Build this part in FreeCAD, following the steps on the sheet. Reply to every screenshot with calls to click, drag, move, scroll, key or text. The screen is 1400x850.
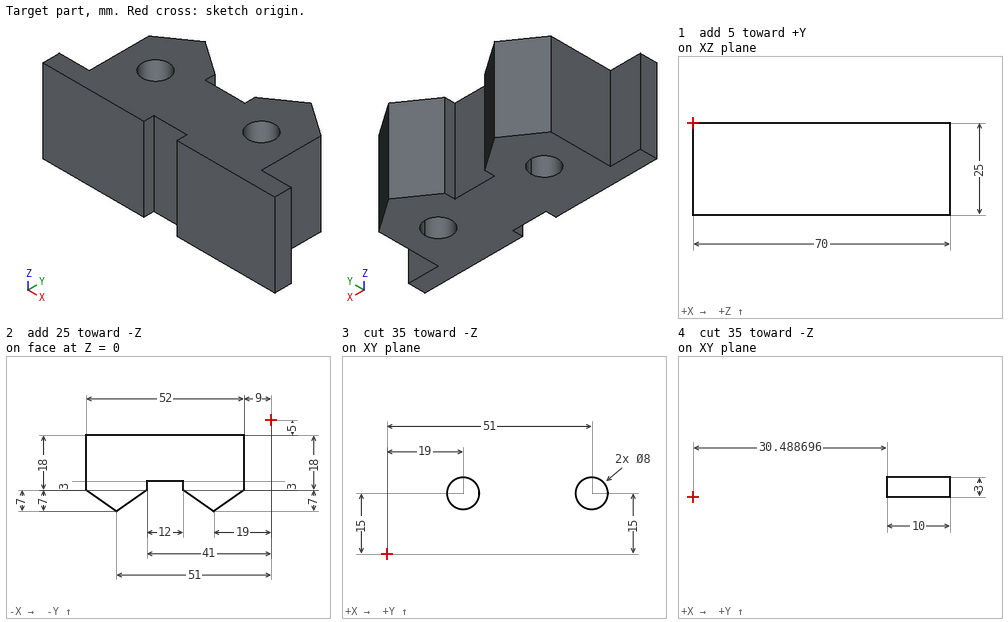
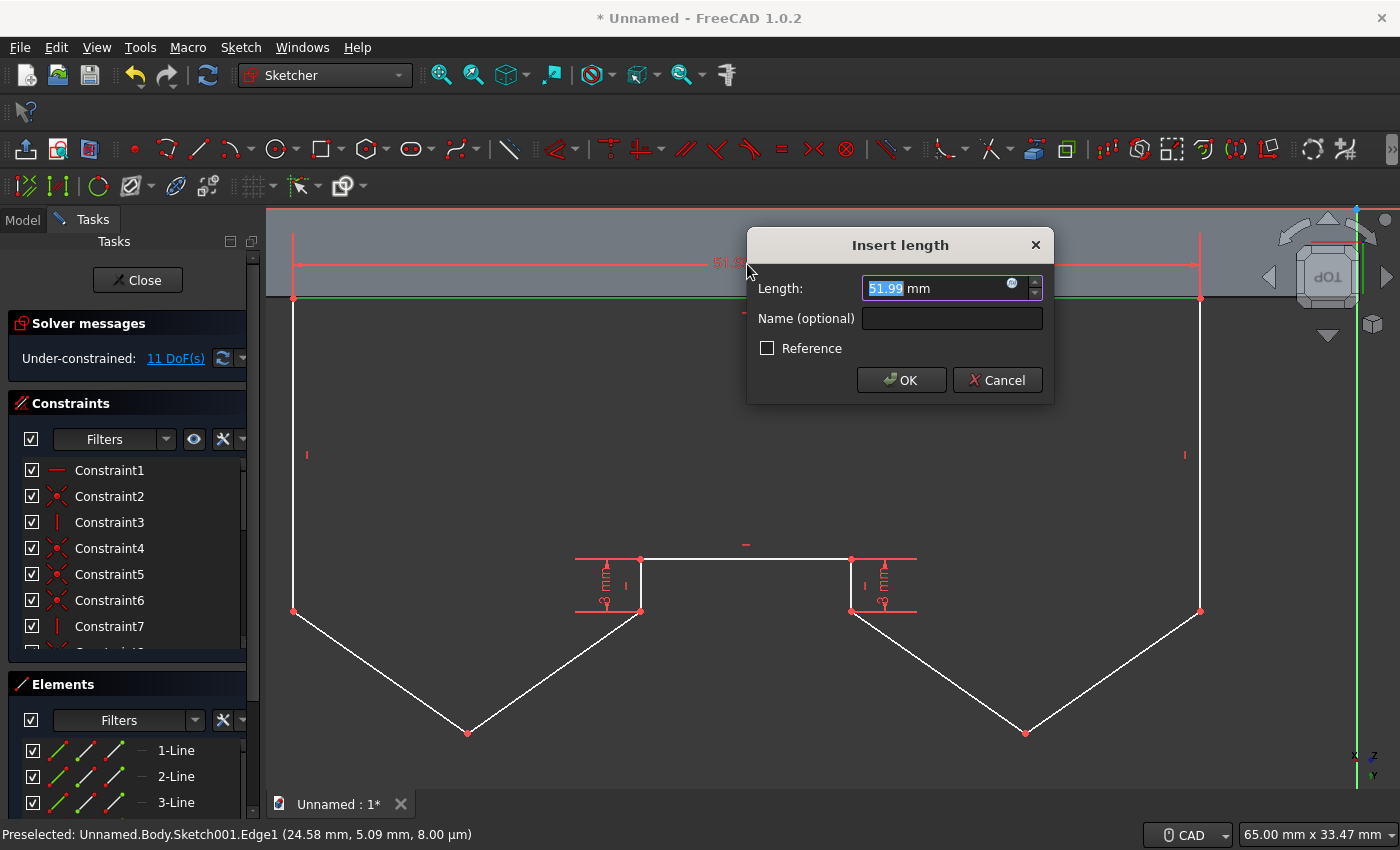
text(52)
key(Return)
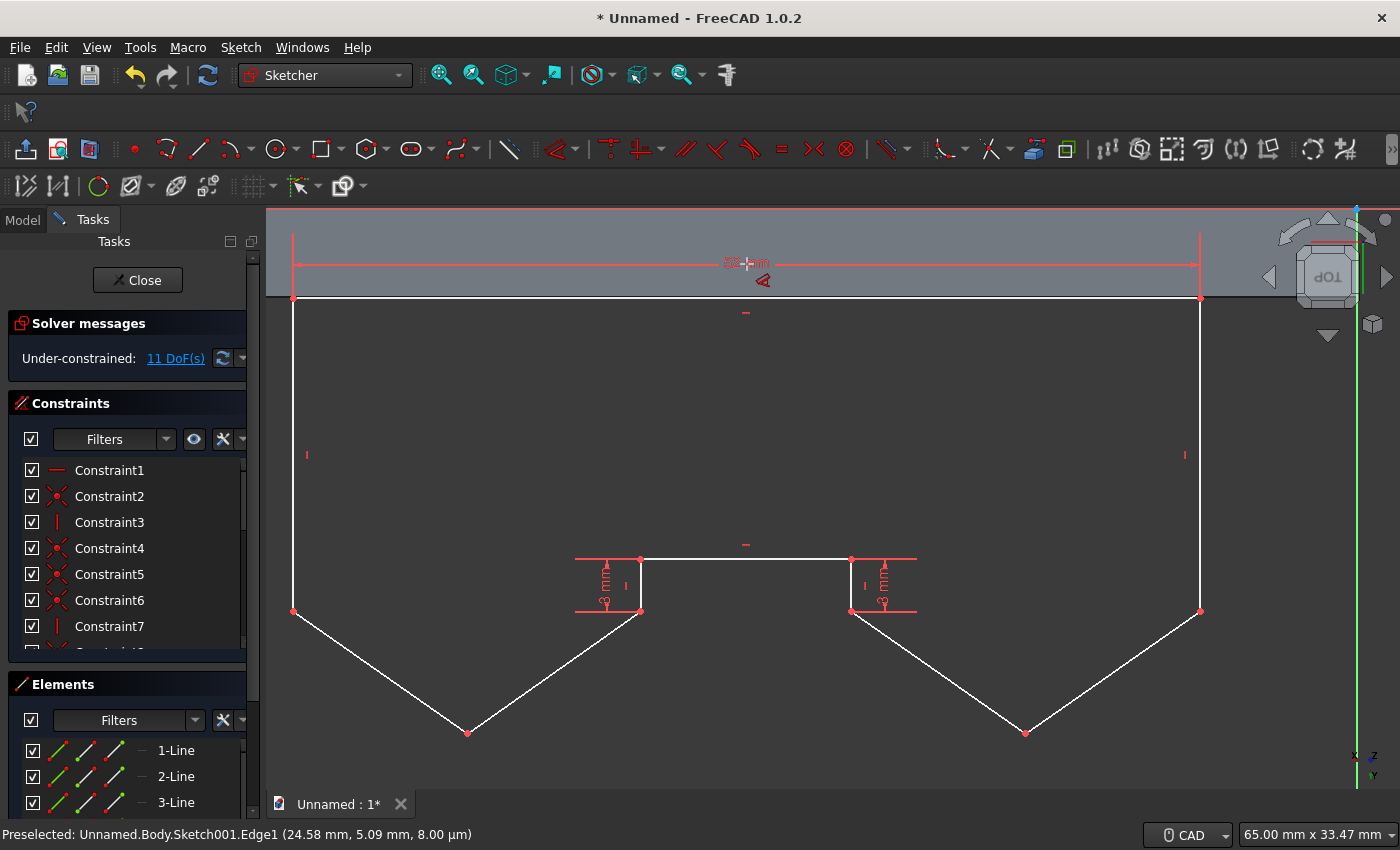
scroll(642, 550, down, 2)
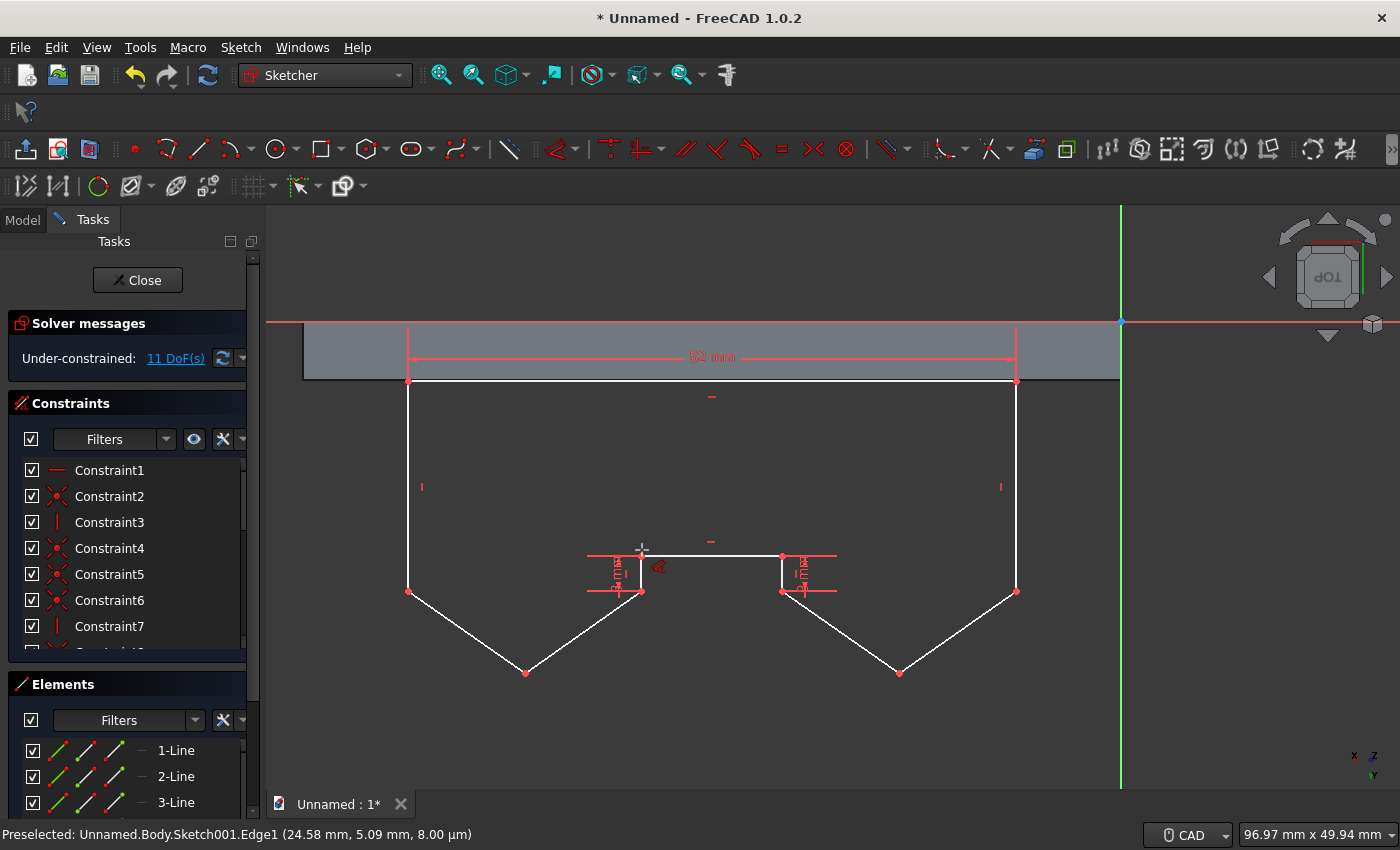
click(408, 444)
click(374, 486)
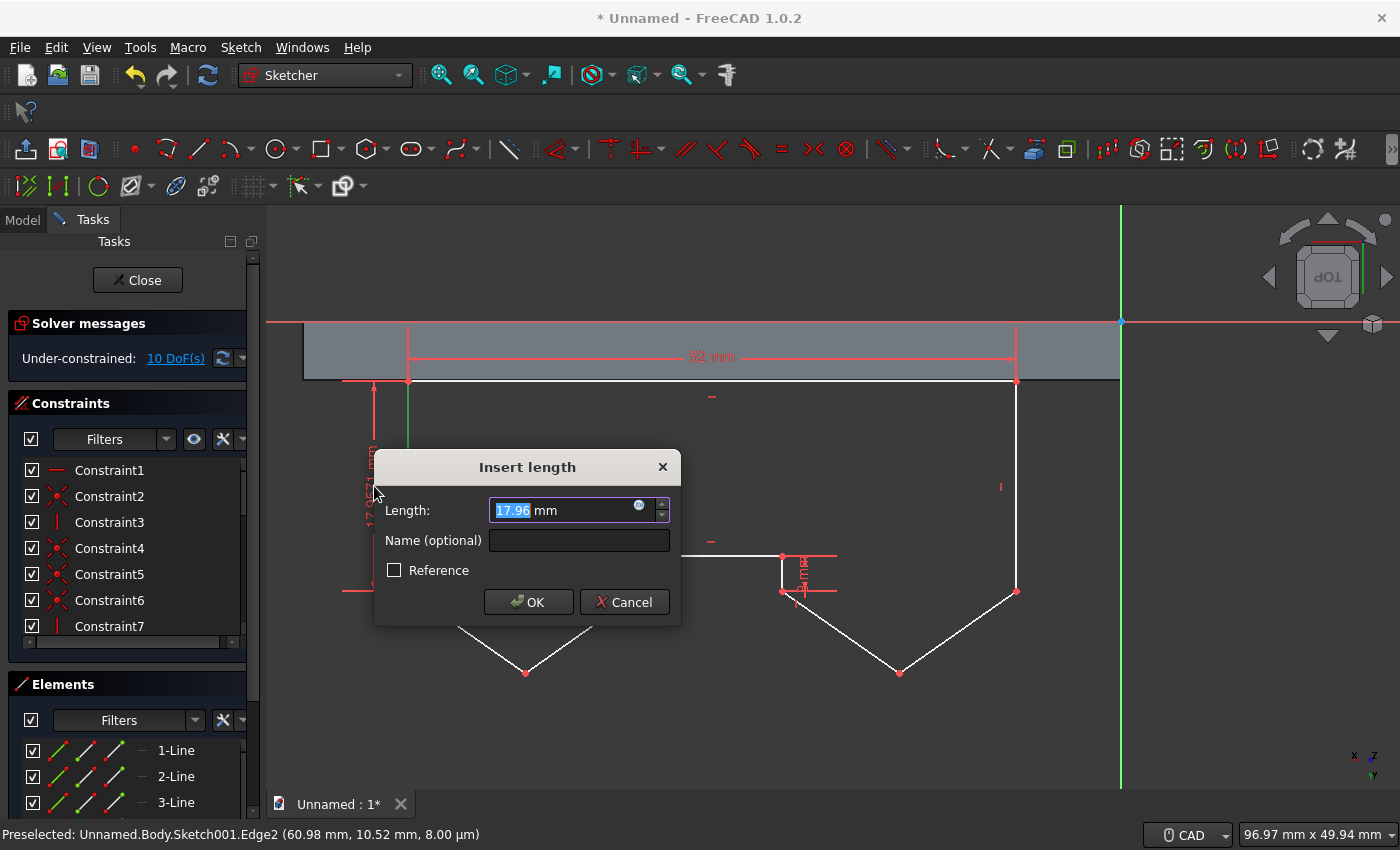
text(18)
key(Return)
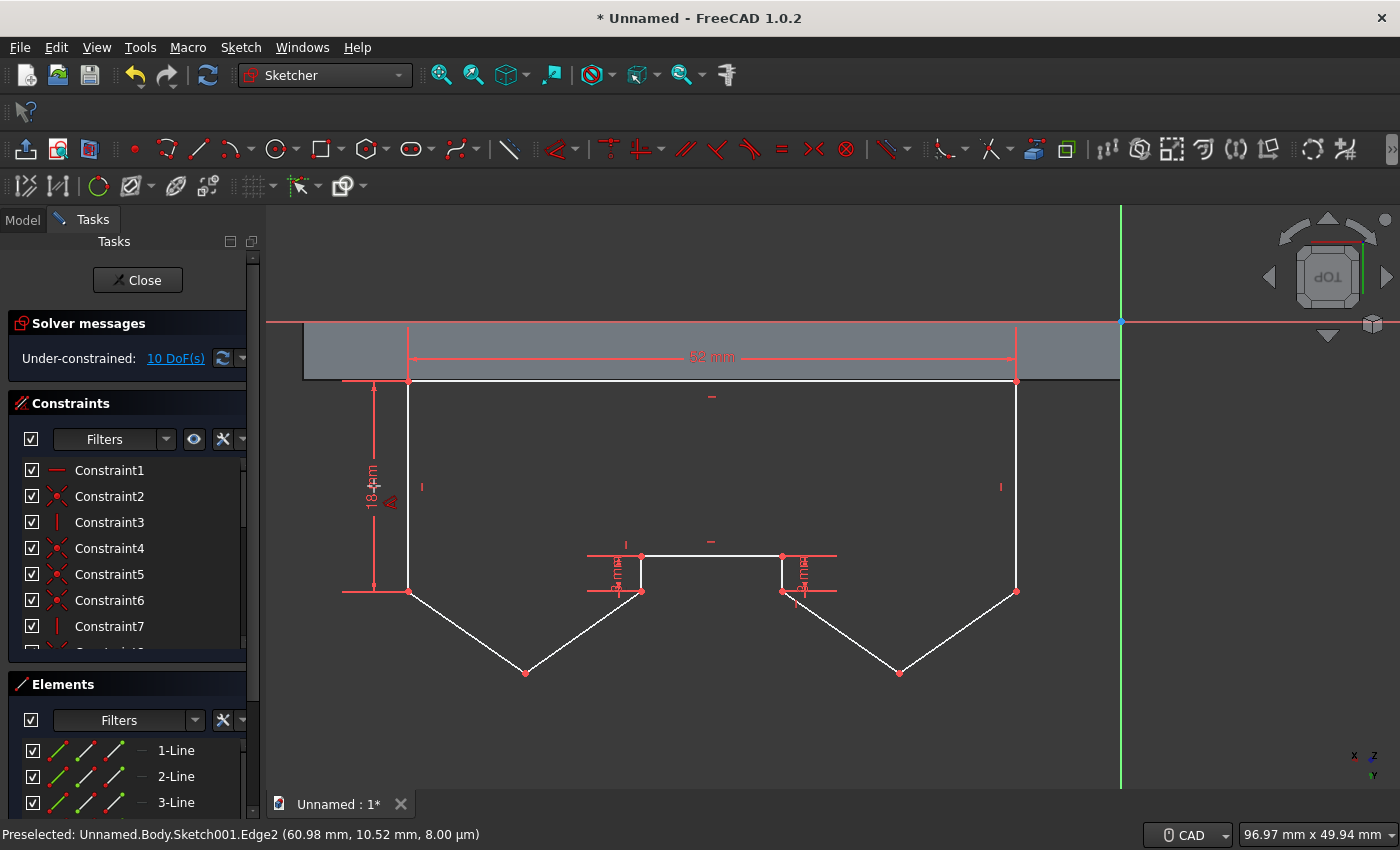
click(684, 556)
click(712, 590)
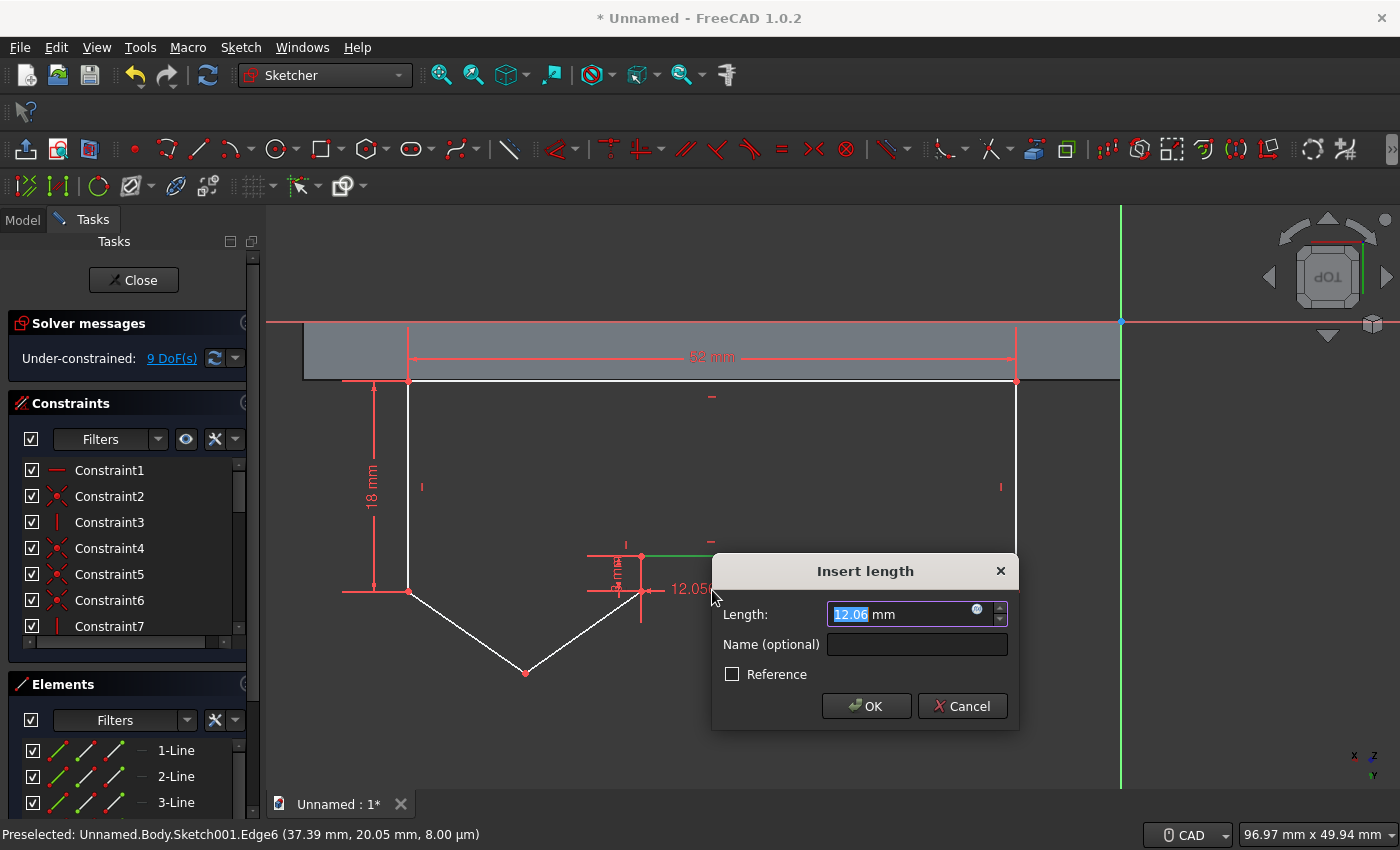
text(12)
key(Return)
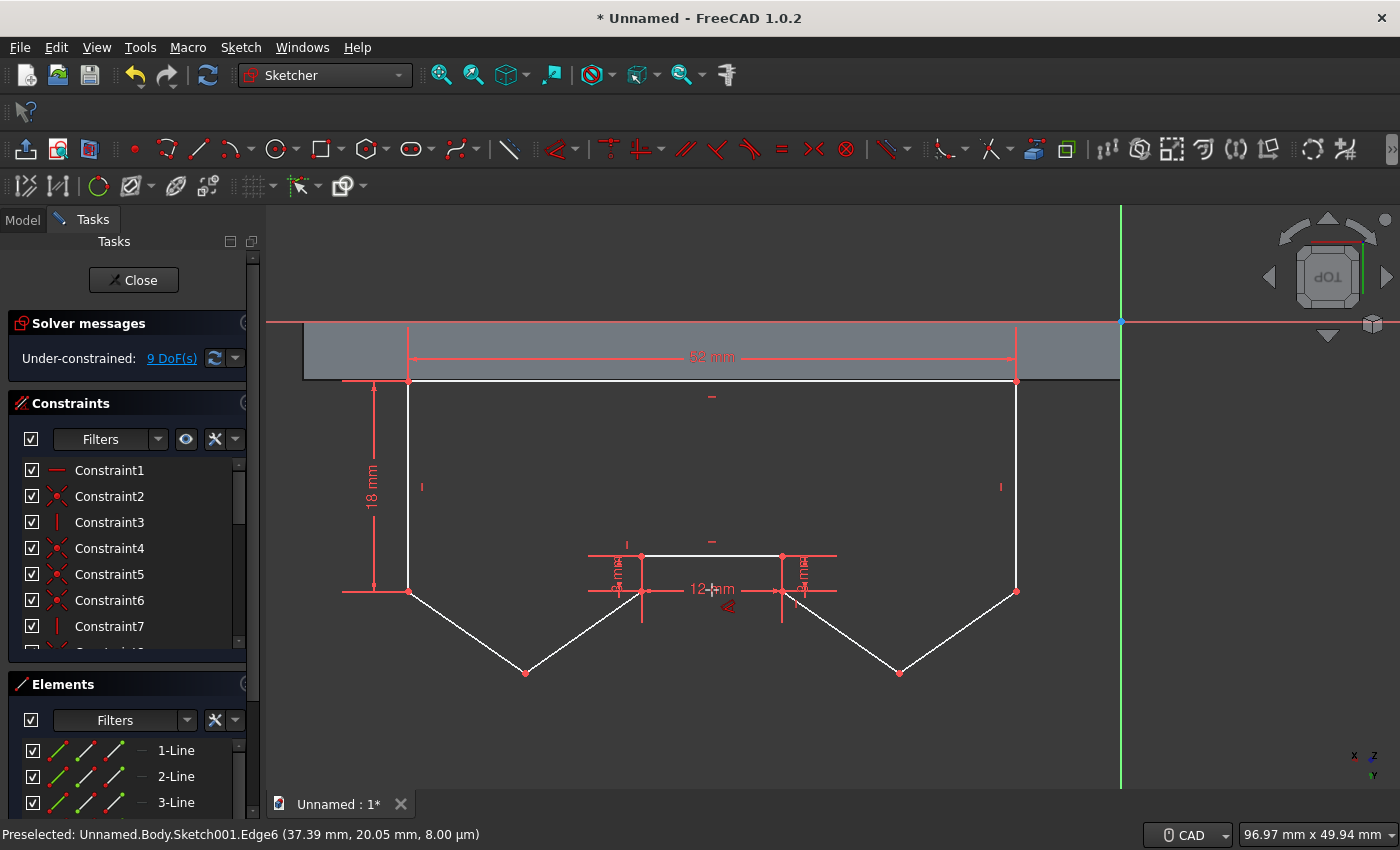
click(1016, 528)
click(1050, 486)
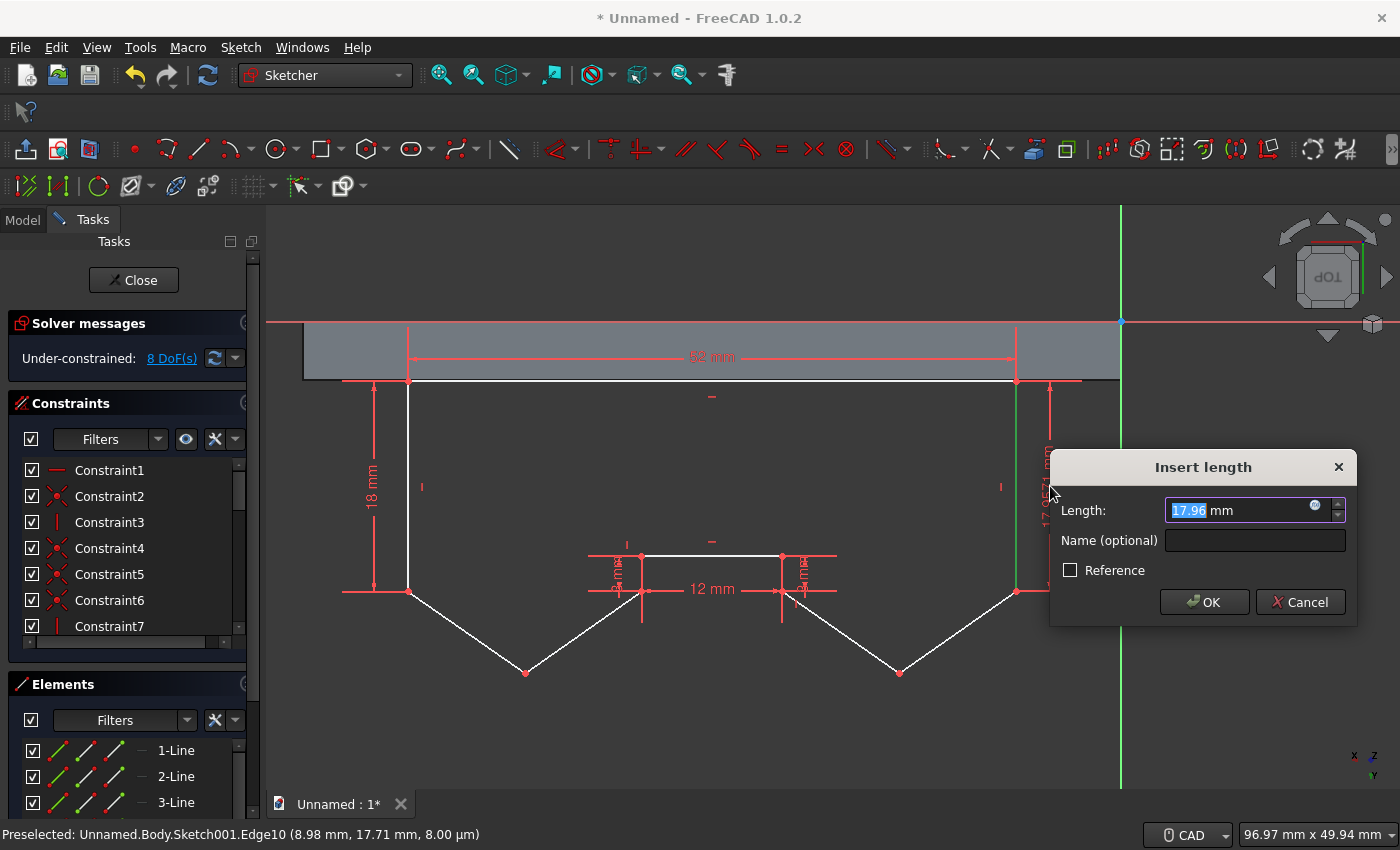
text(18)
key(Return)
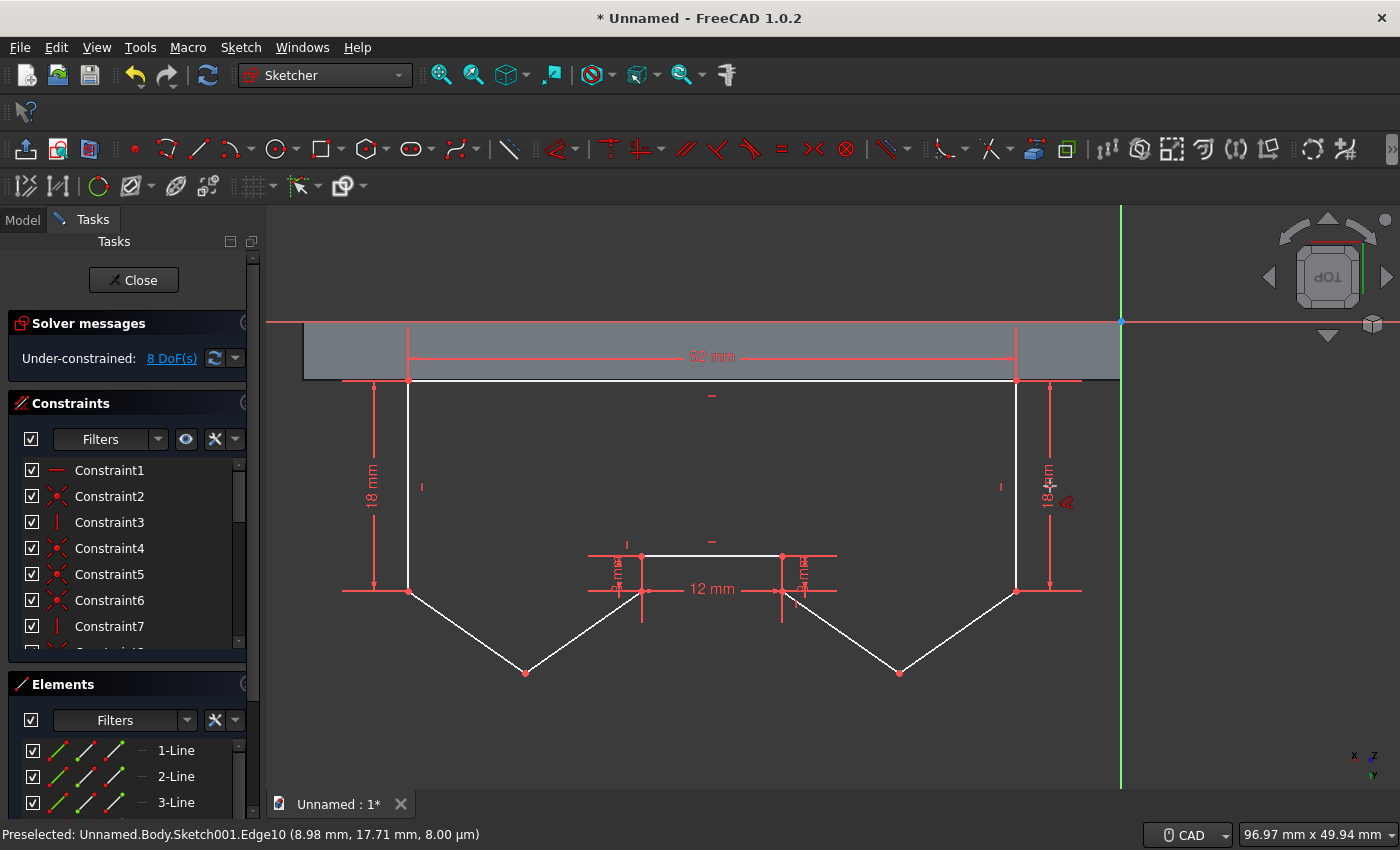
click(1016, 381)
click(1069, 288)